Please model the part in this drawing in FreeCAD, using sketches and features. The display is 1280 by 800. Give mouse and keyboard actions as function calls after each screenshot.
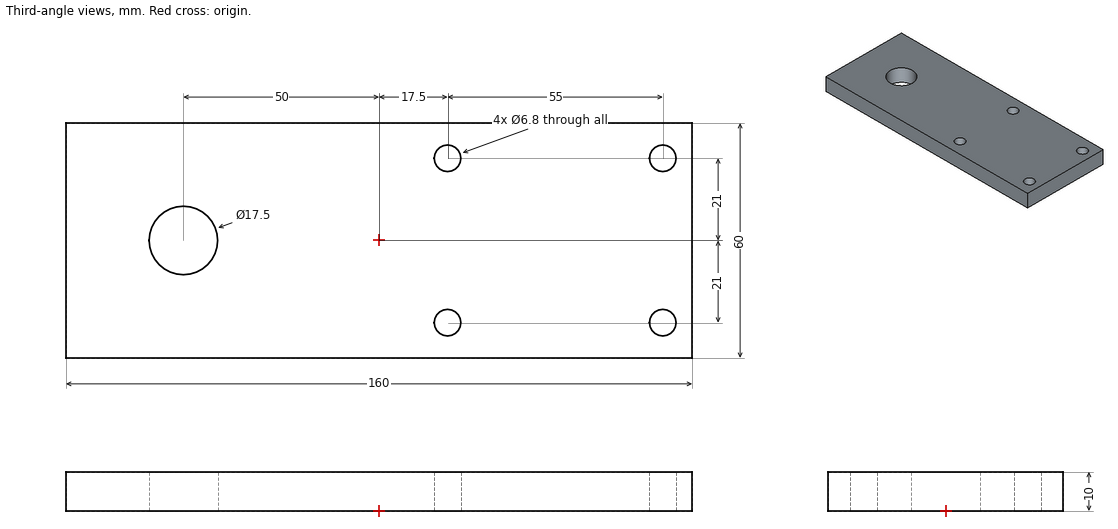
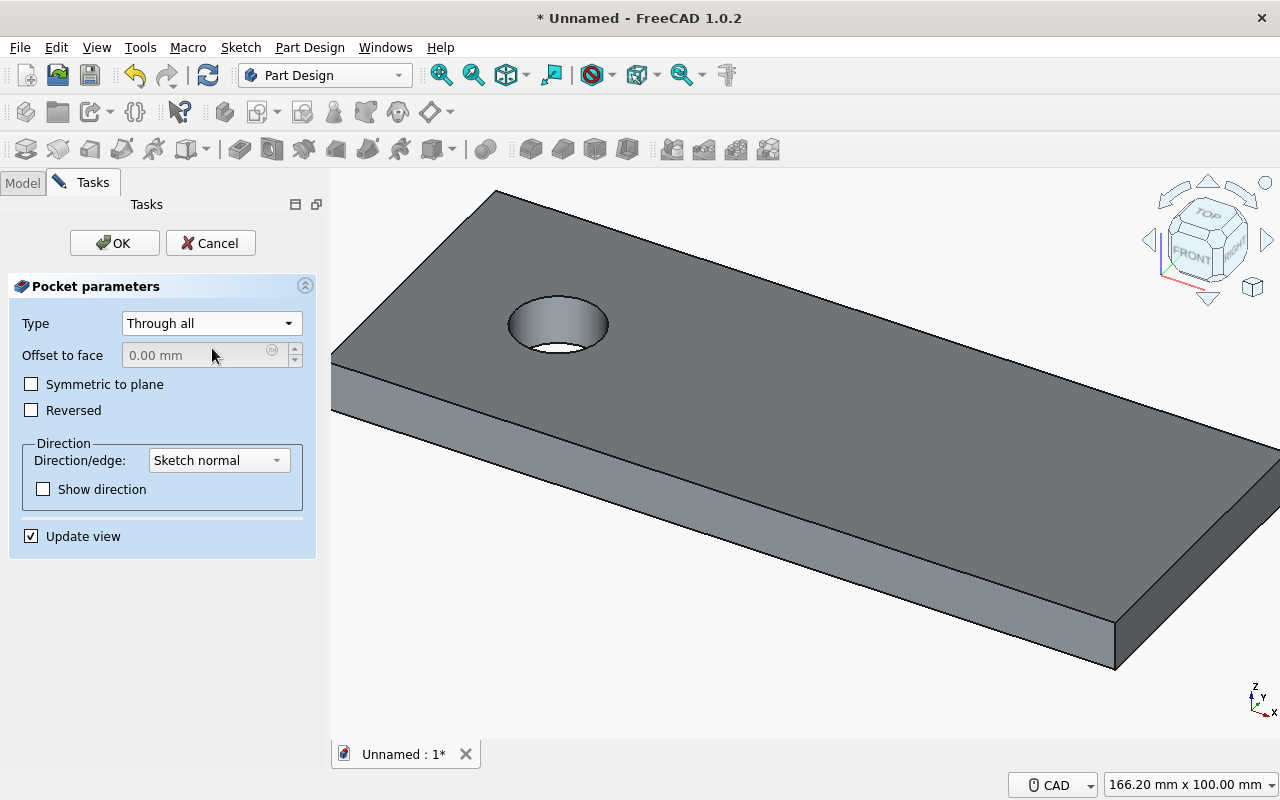
click(115, 243)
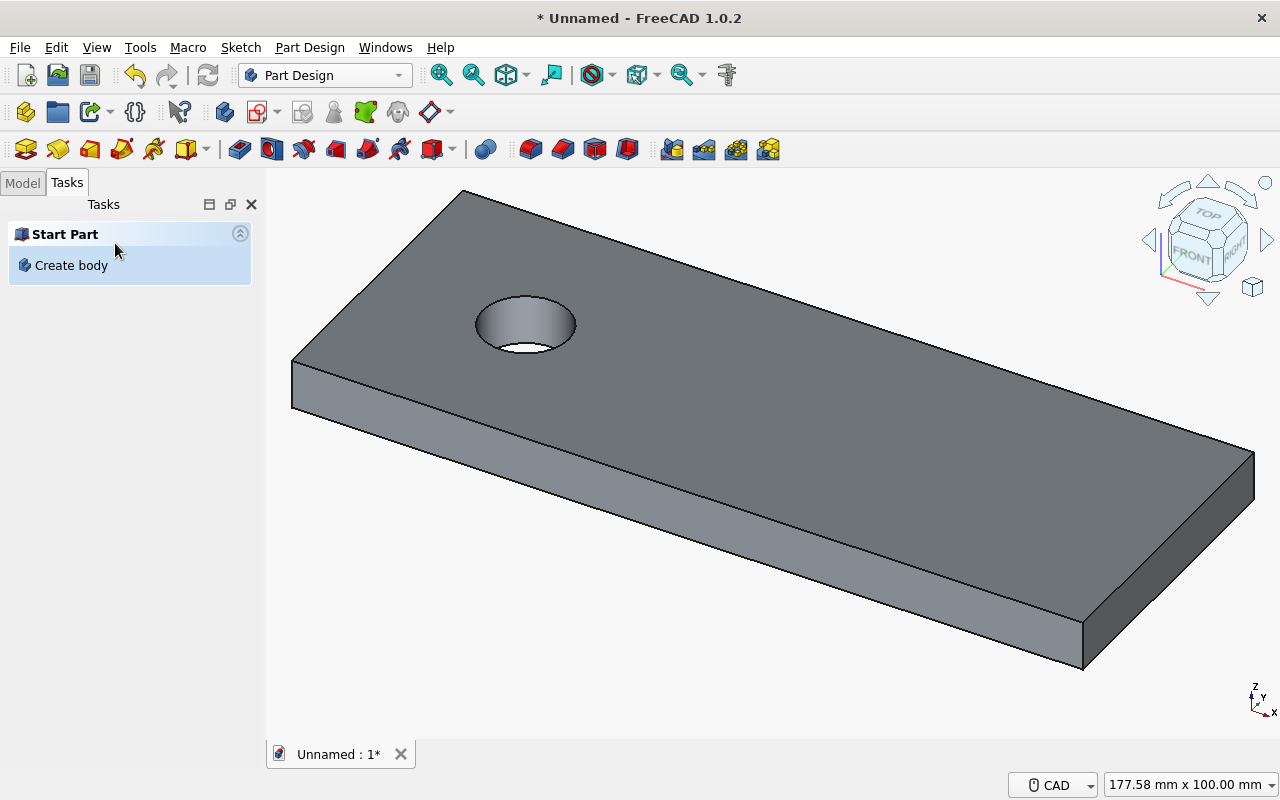
click(999, 481)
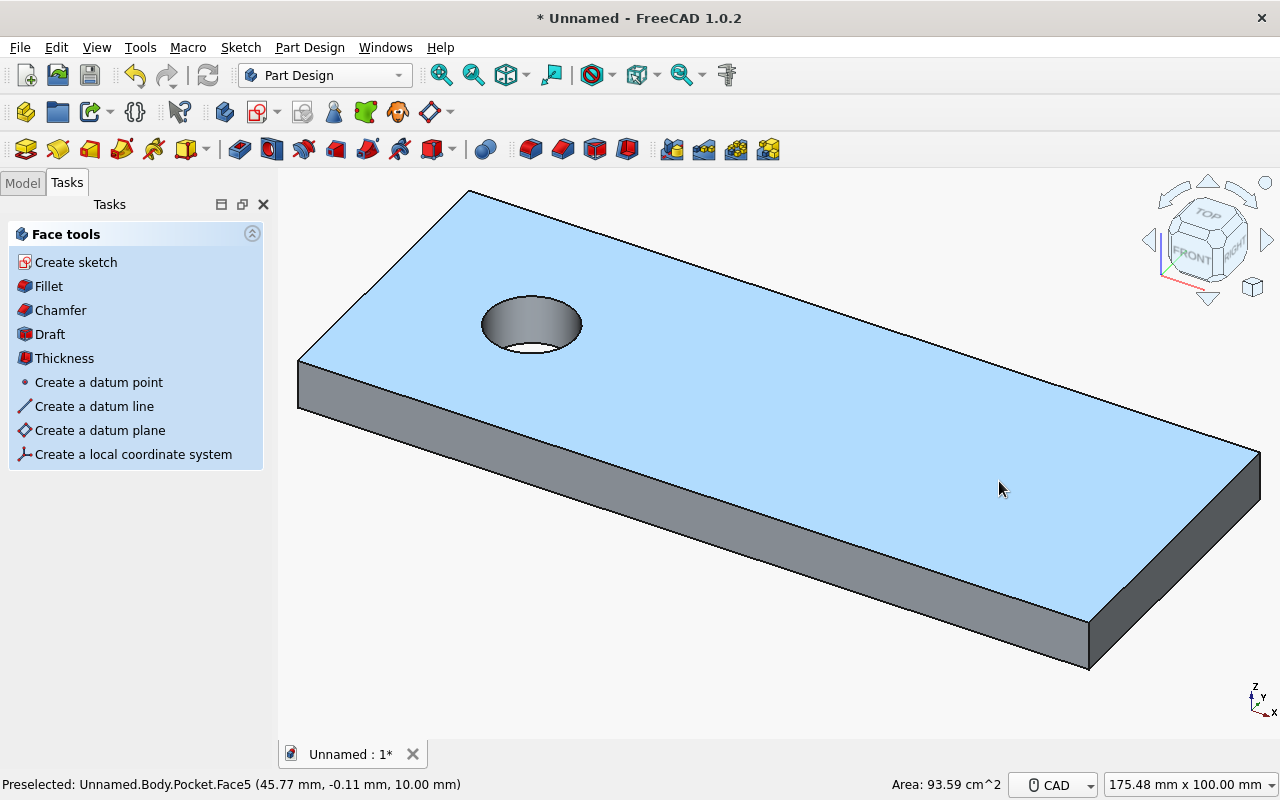
click(258, 112)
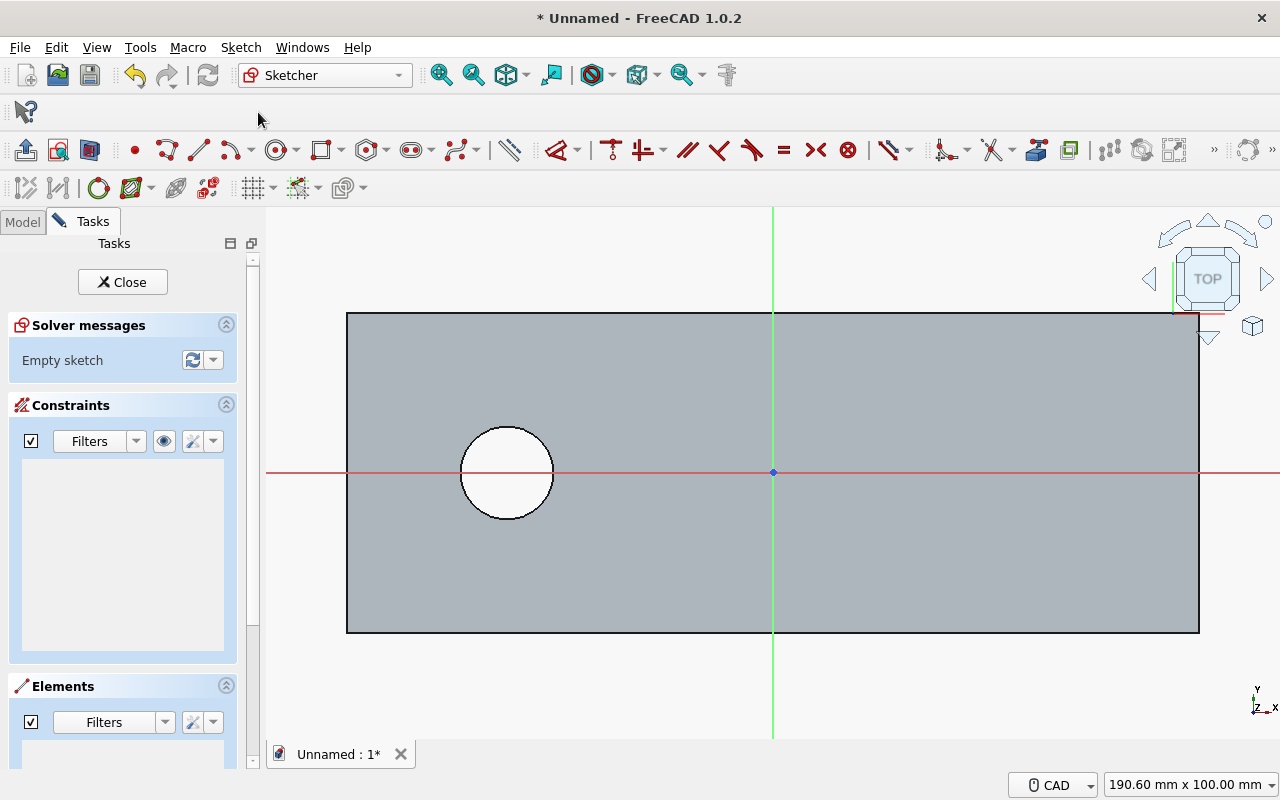
scroll(294, 473, down, 1)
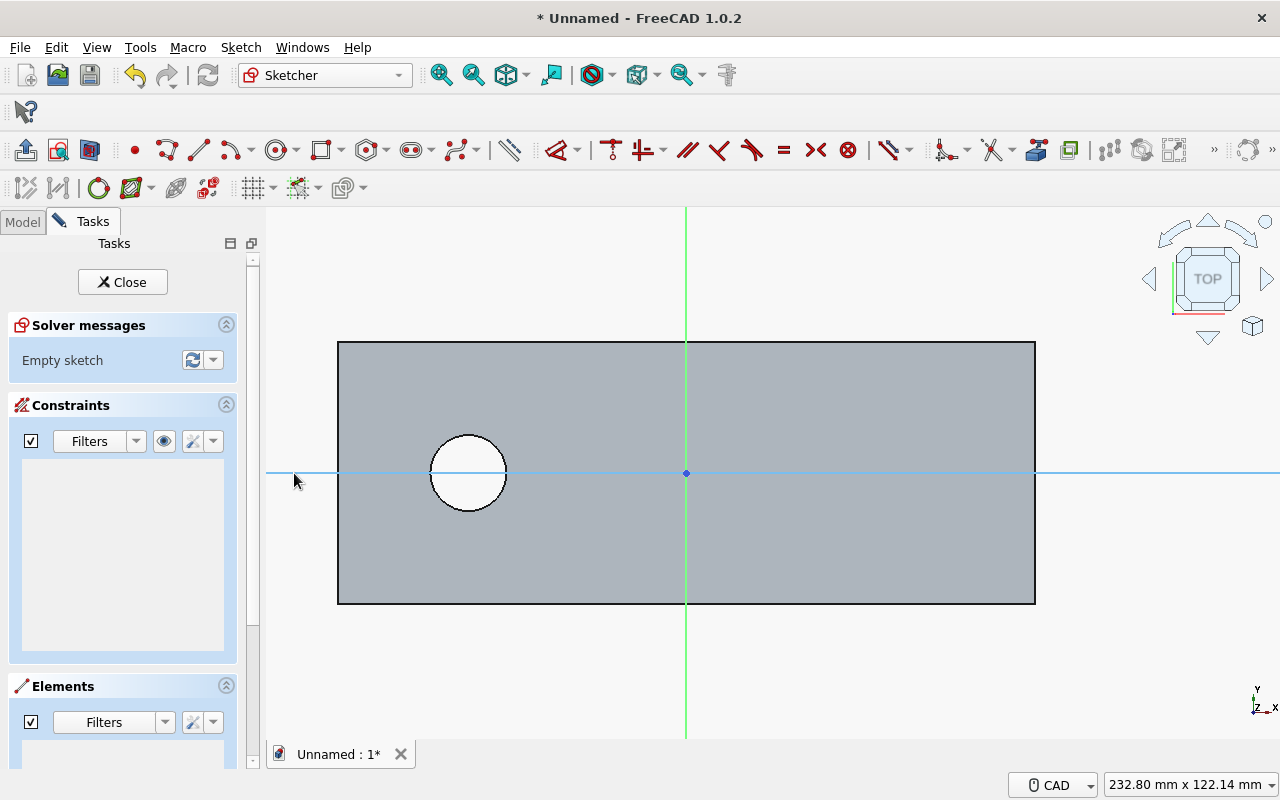
scroll(1115, 473, up, 2)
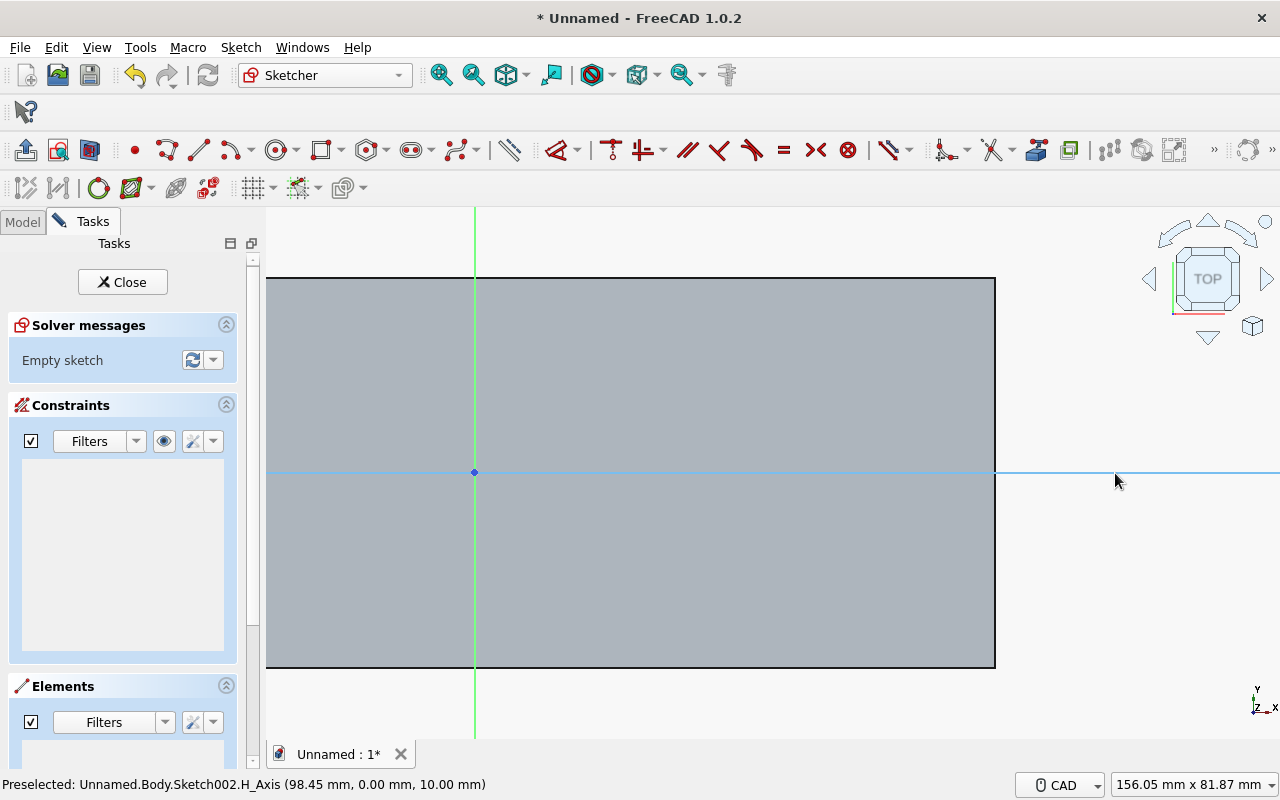
key(g)
key(c)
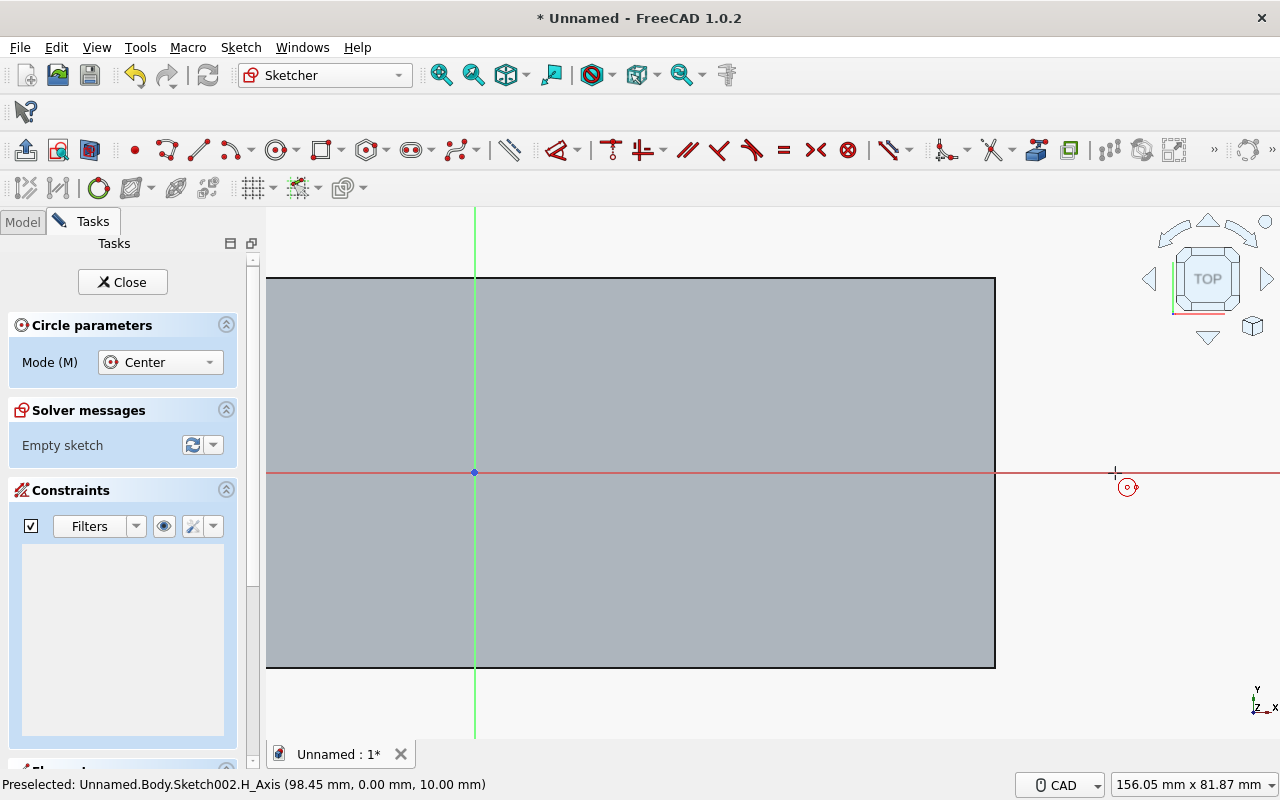
click(589, 336)
click(604, 321)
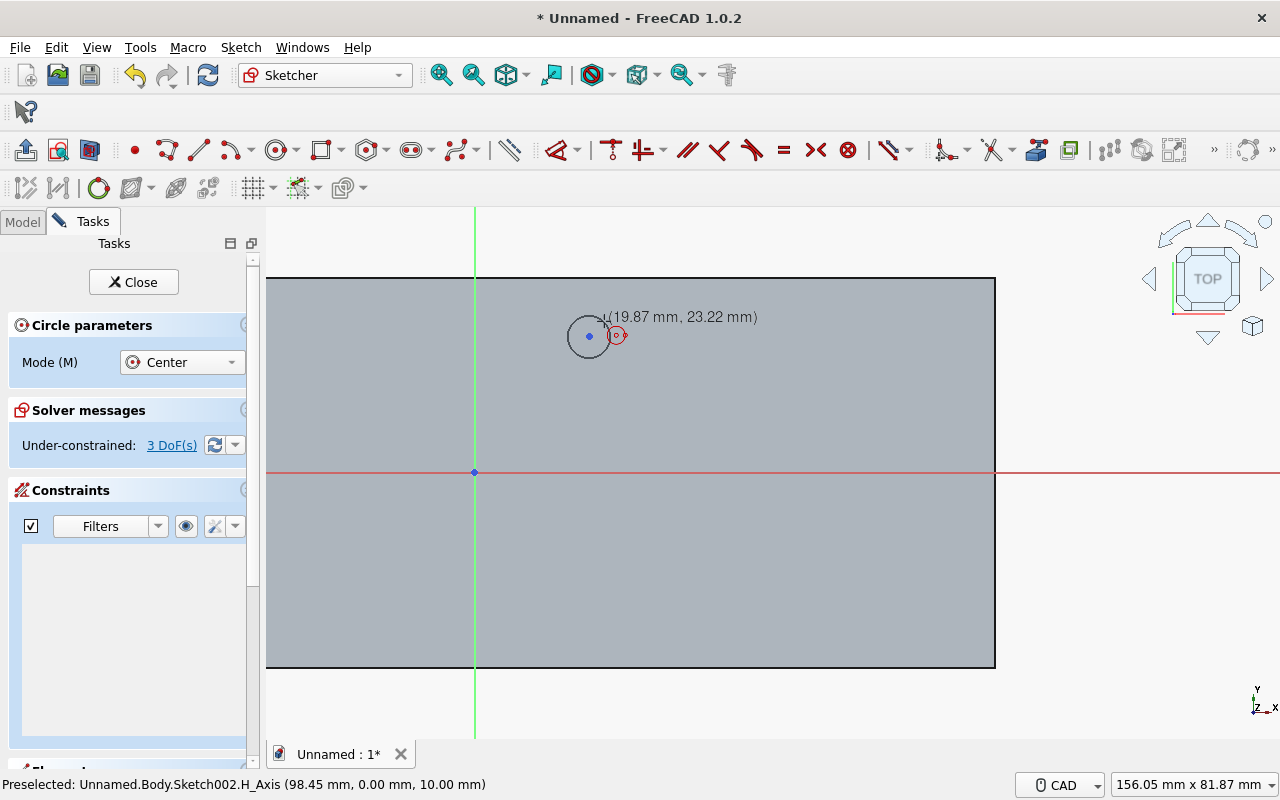
click(946, 336)
click(962, 321)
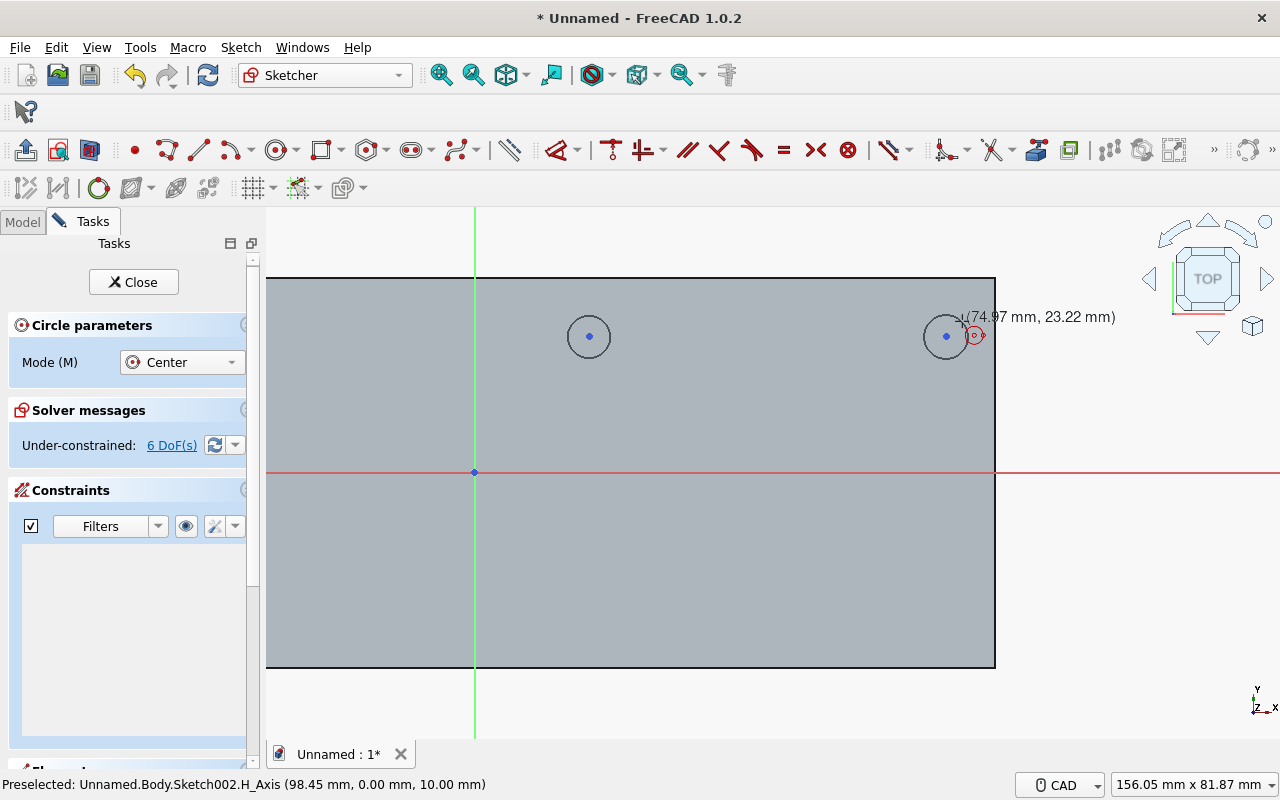
click(589, 609)
click(604, 594)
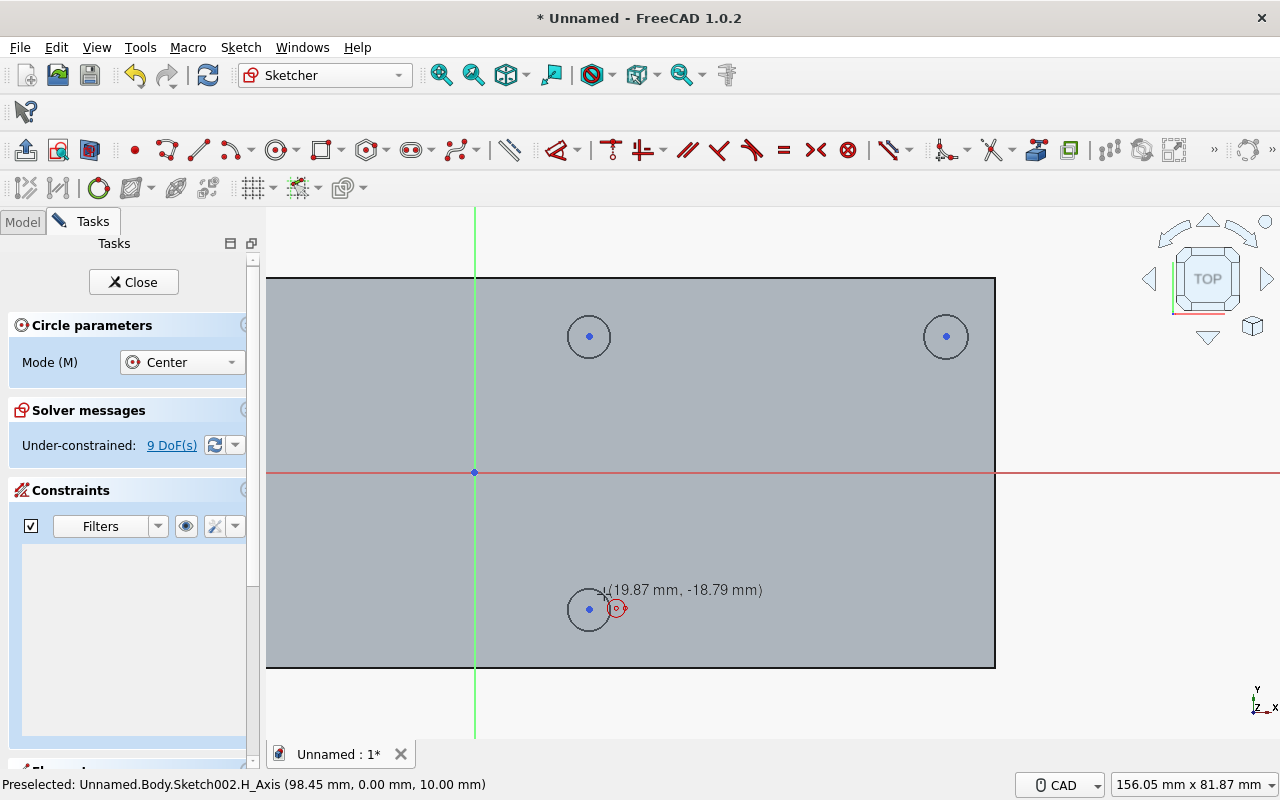
click(946, 609)
click(962, 594)
key(Escape)